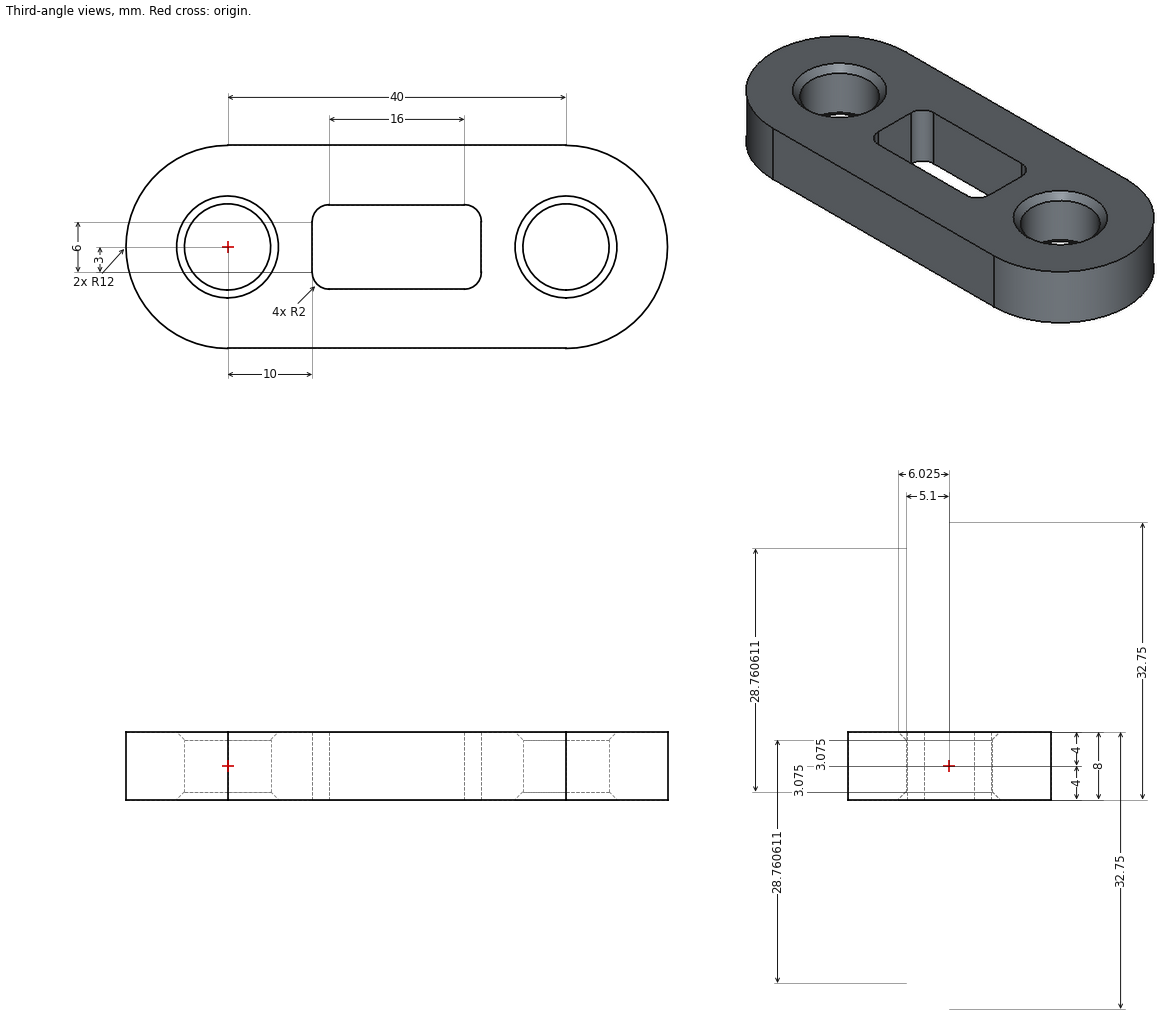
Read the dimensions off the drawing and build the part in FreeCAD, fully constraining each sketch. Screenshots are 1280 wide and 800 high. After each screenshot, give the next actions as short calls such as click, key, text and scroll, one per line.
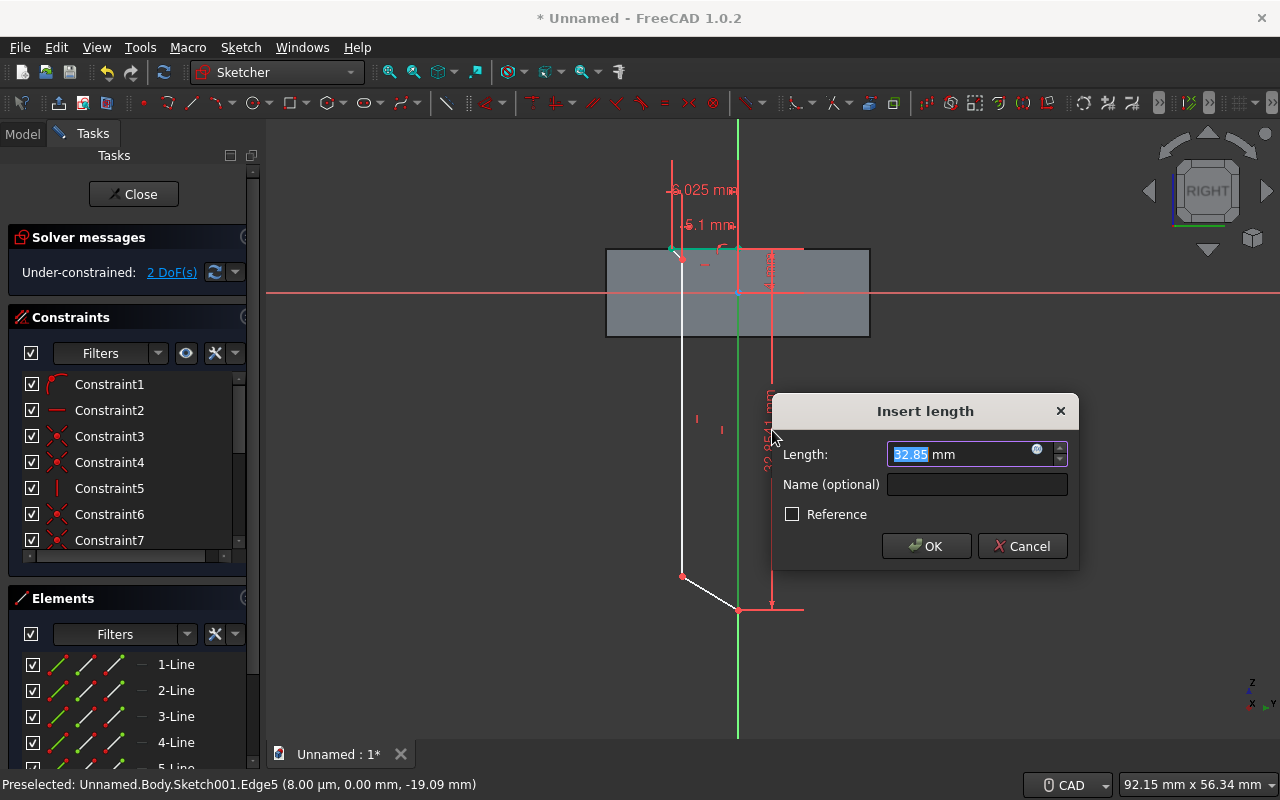
text(32.75)
key(Return)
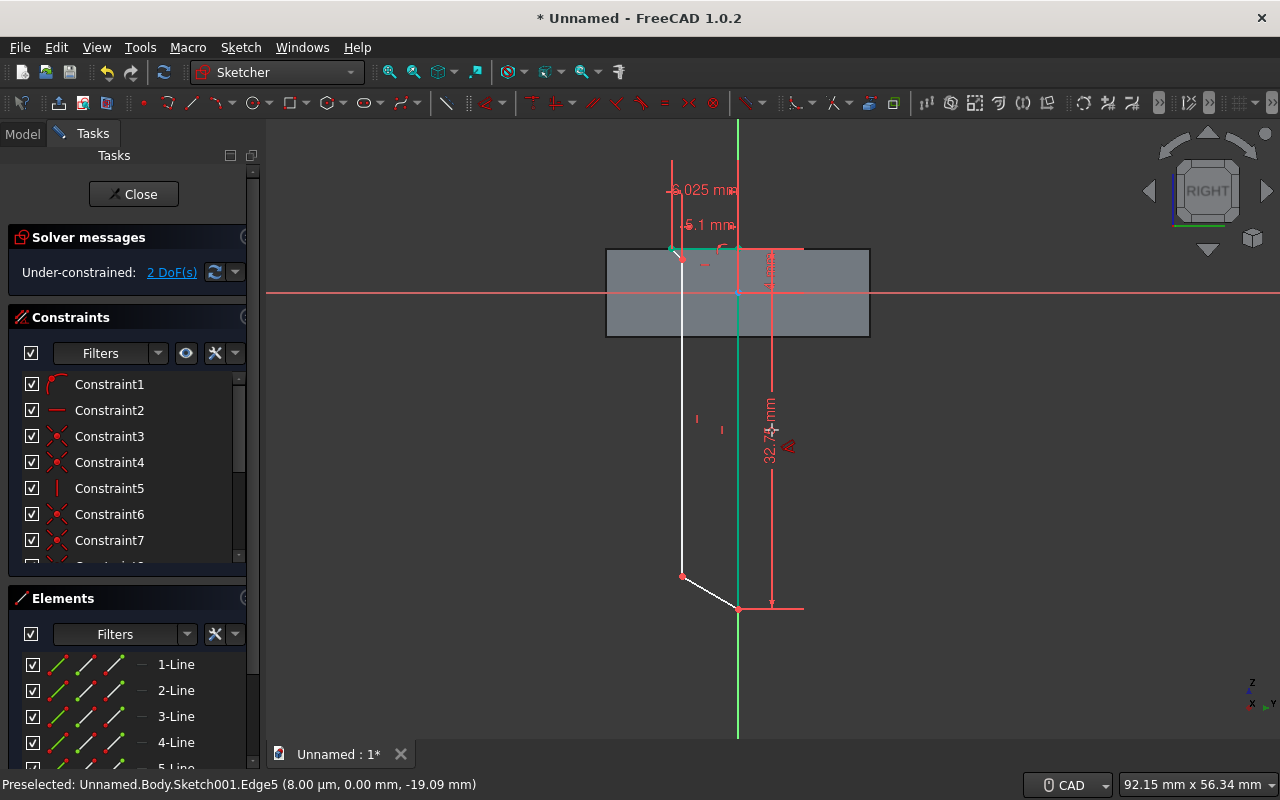
click(682, 260)
click(648, 276)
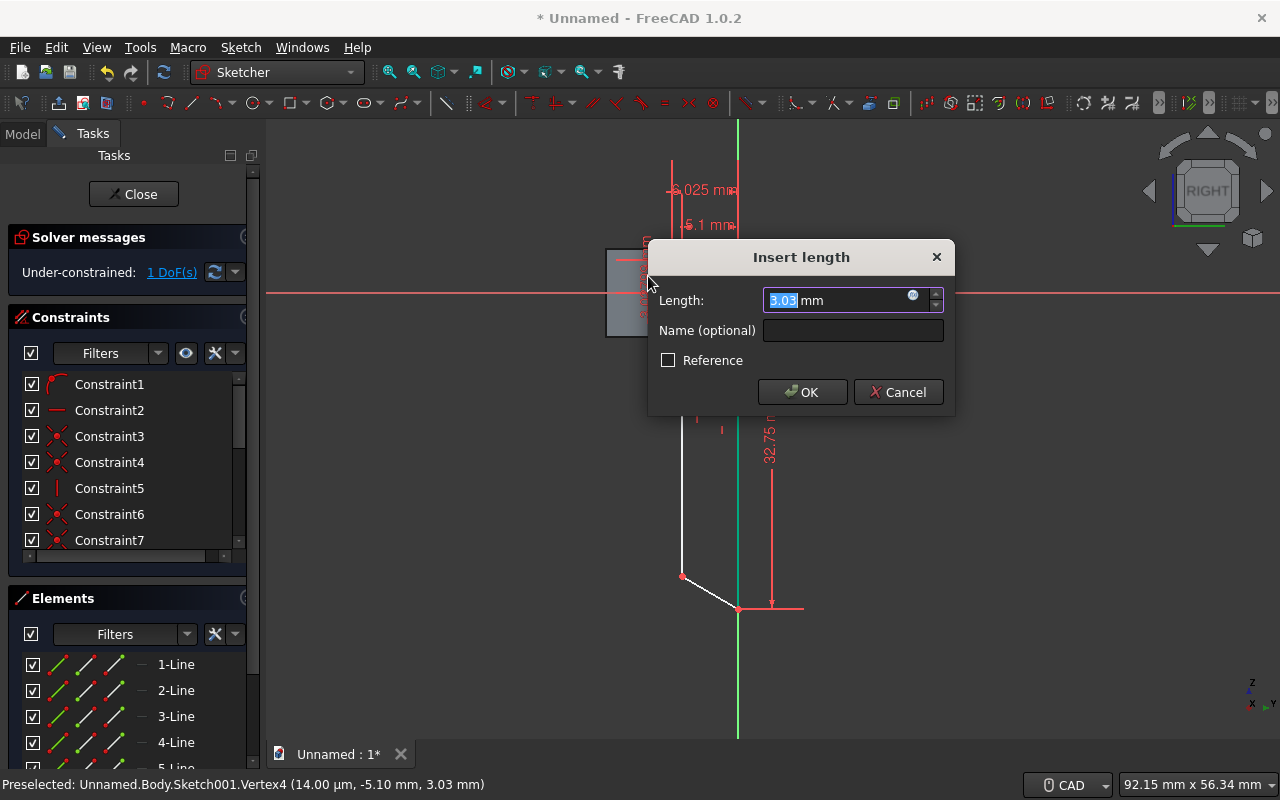
text(3.075)
key(Return)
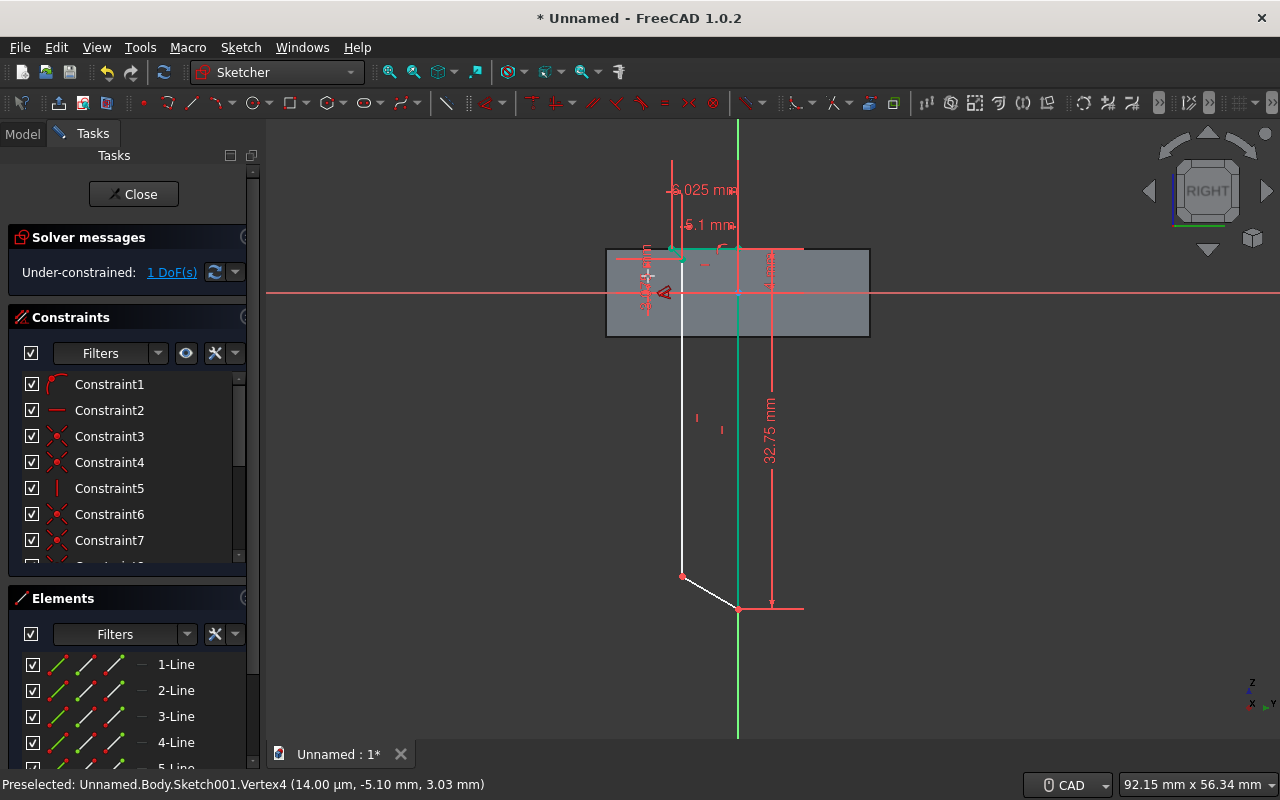
click(682, 354)
click(648, 418)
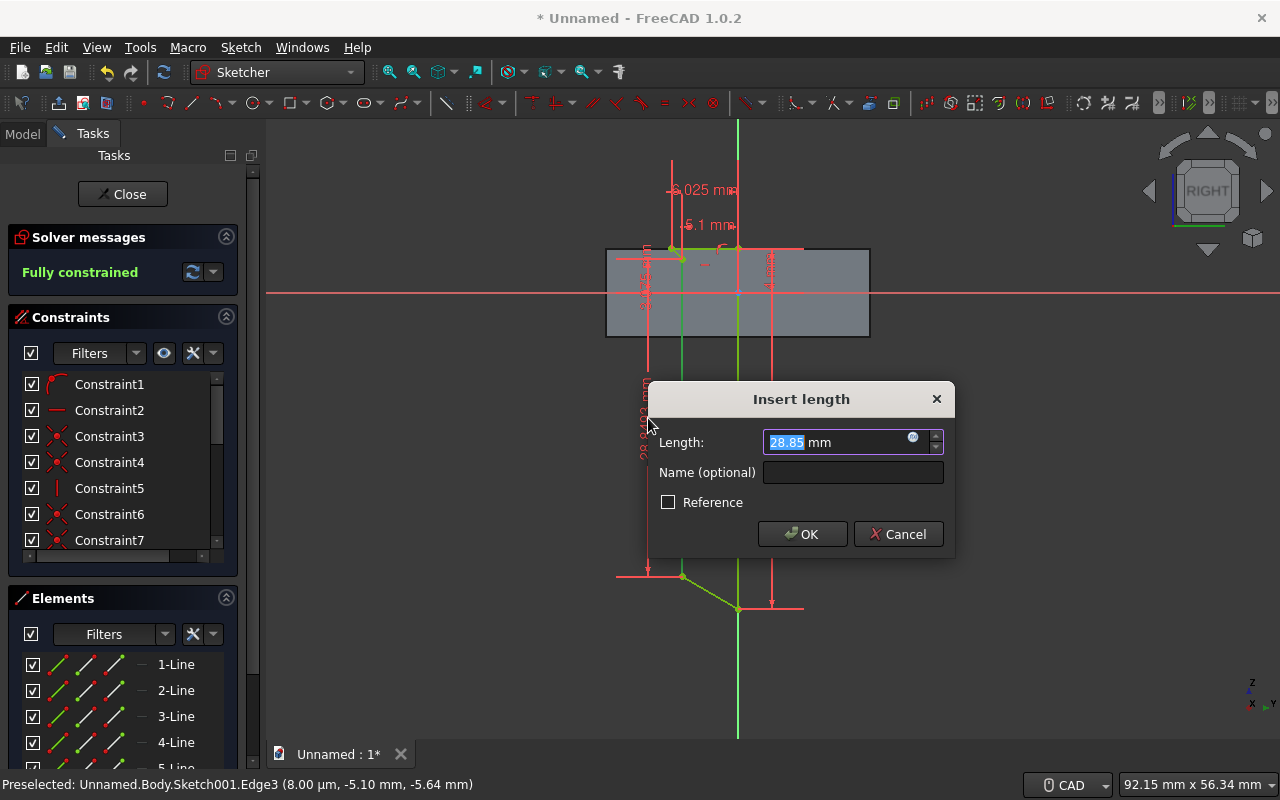
text(28.760611)
key(Return)
key(Escape)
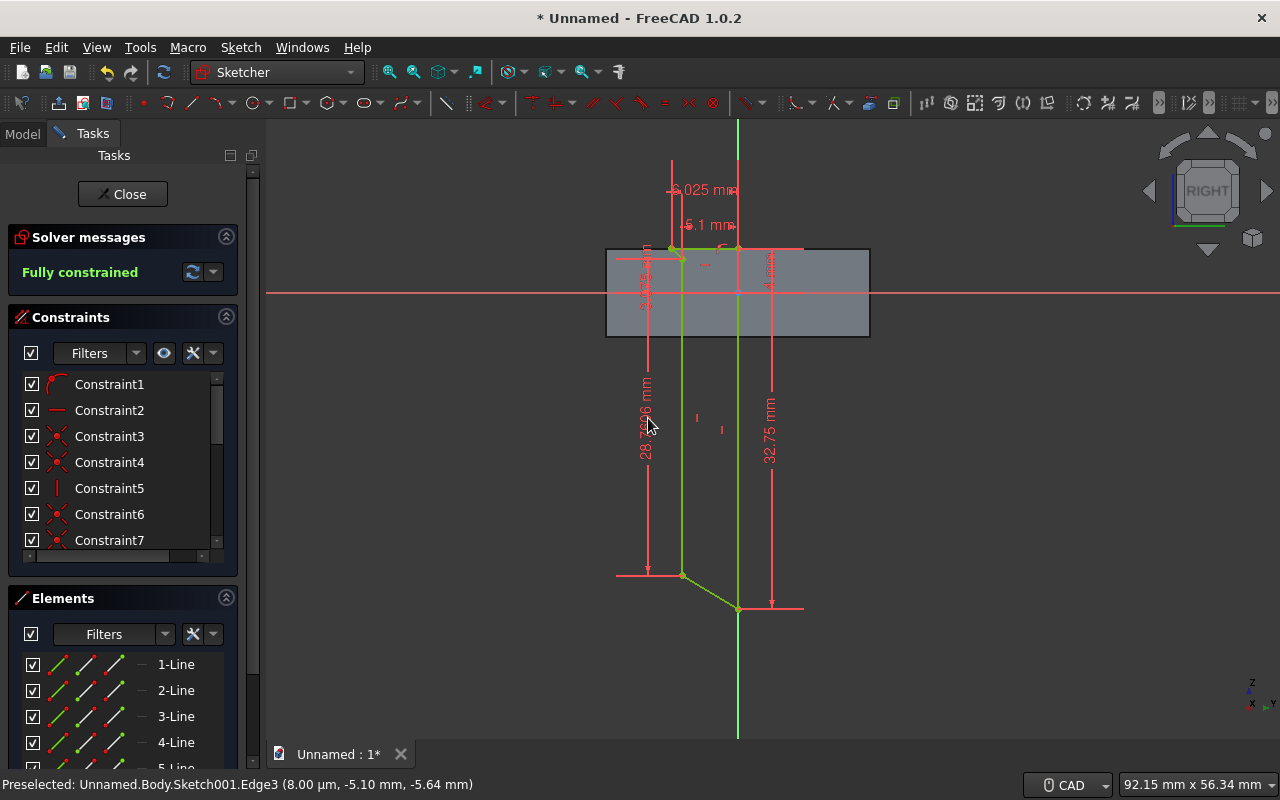
click(123, 194)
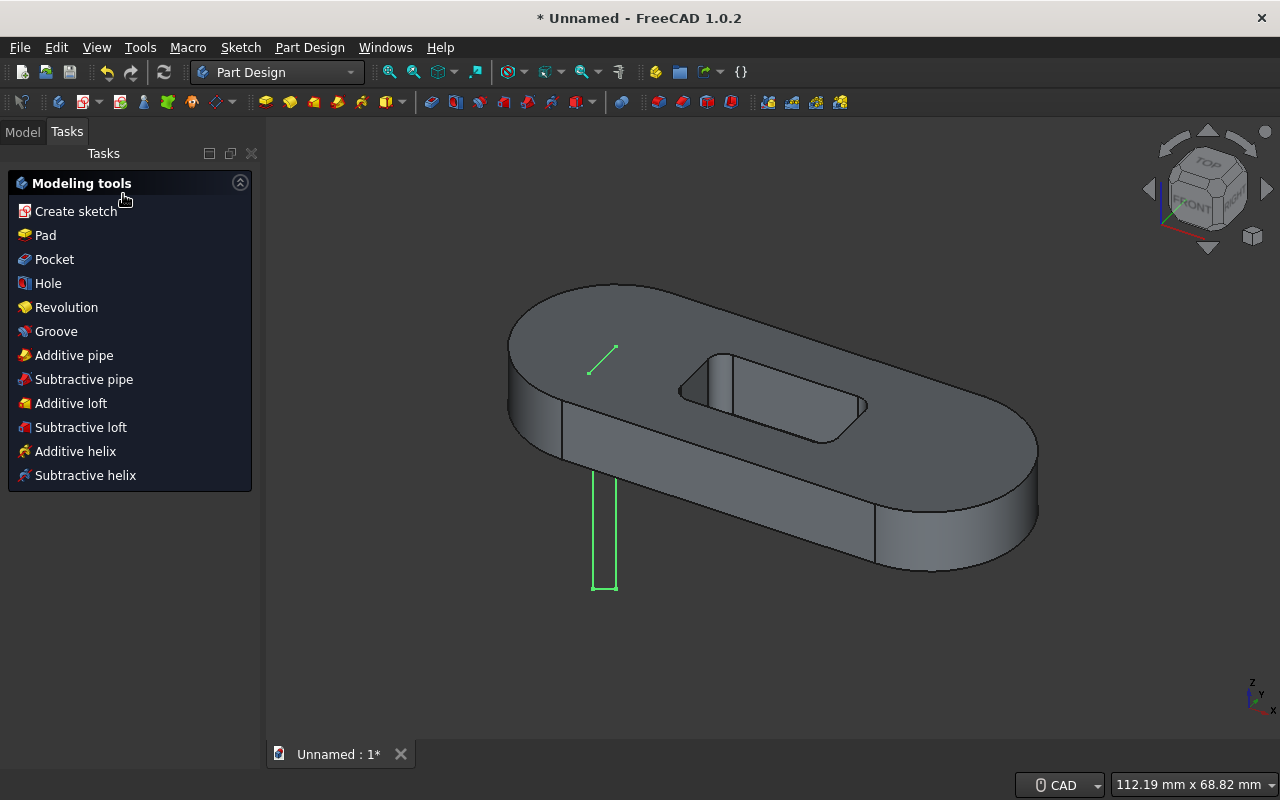
click(480, 102)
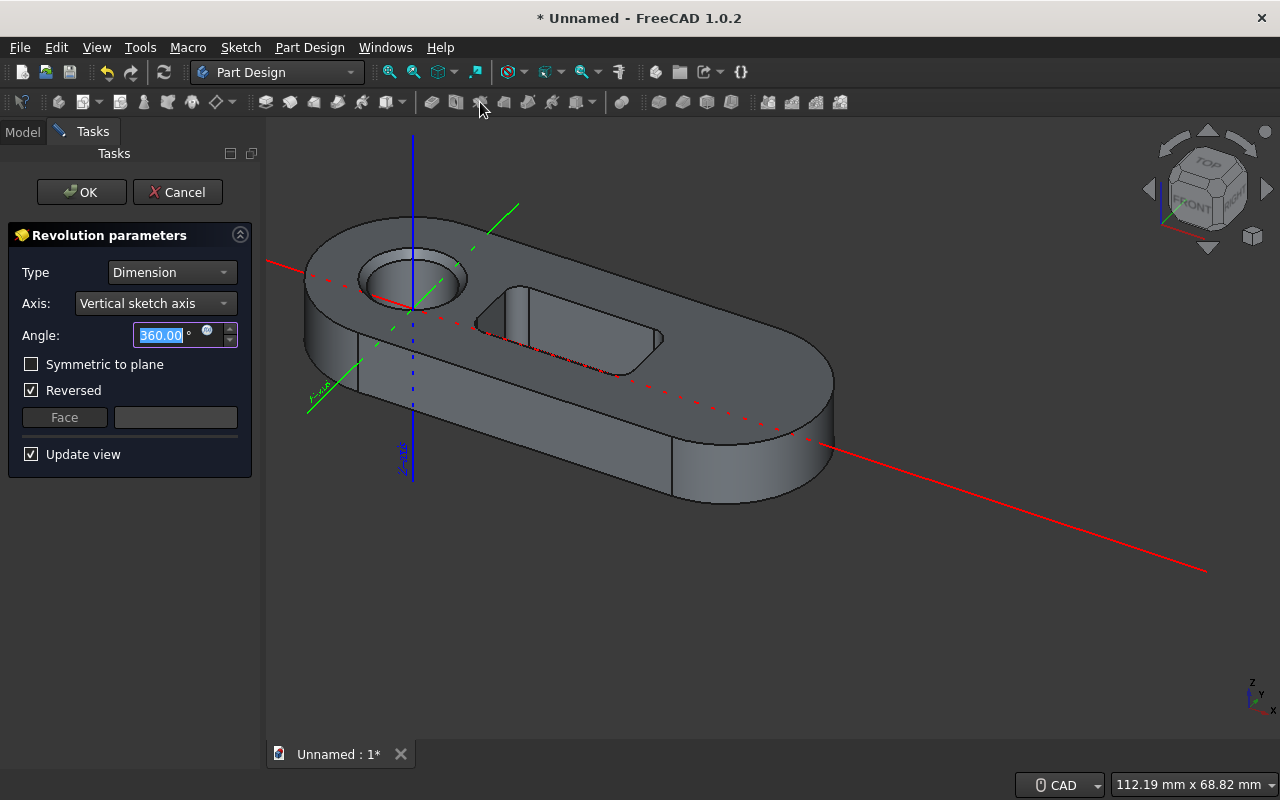
click(82, 192)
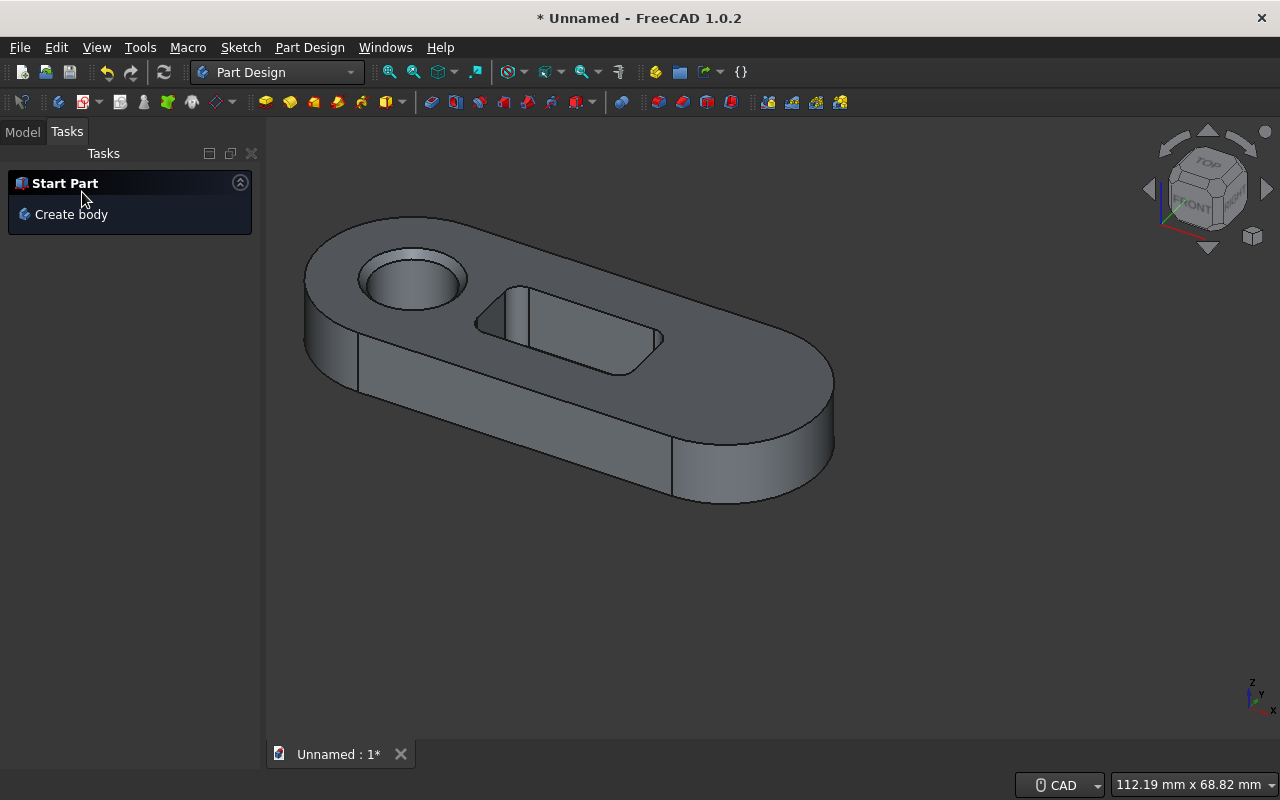
key(v)
key(f)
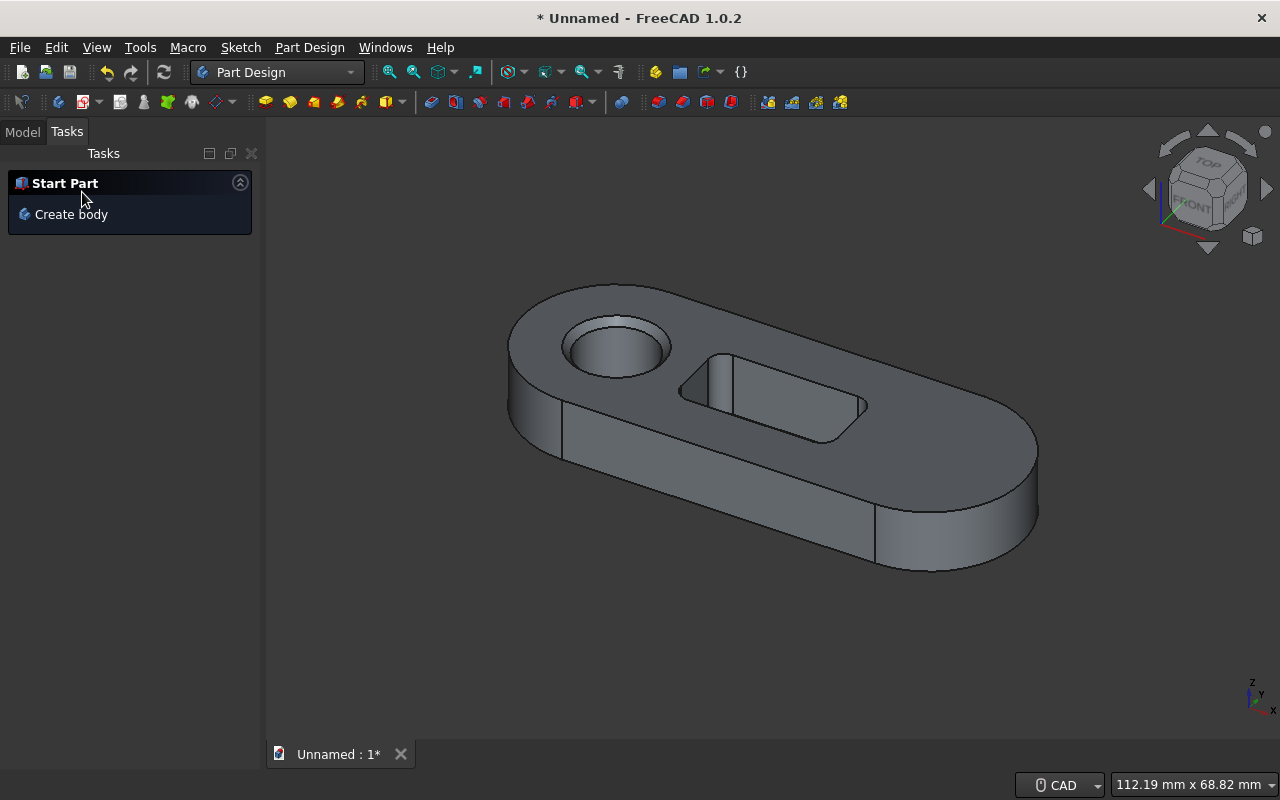
click(23, 131)